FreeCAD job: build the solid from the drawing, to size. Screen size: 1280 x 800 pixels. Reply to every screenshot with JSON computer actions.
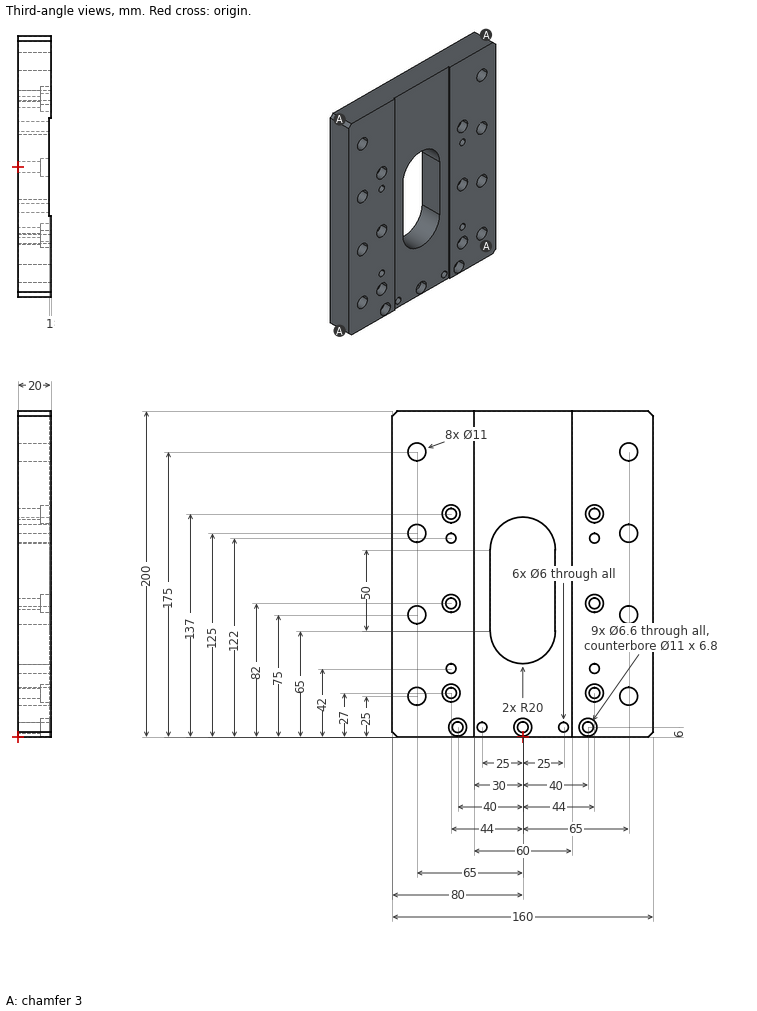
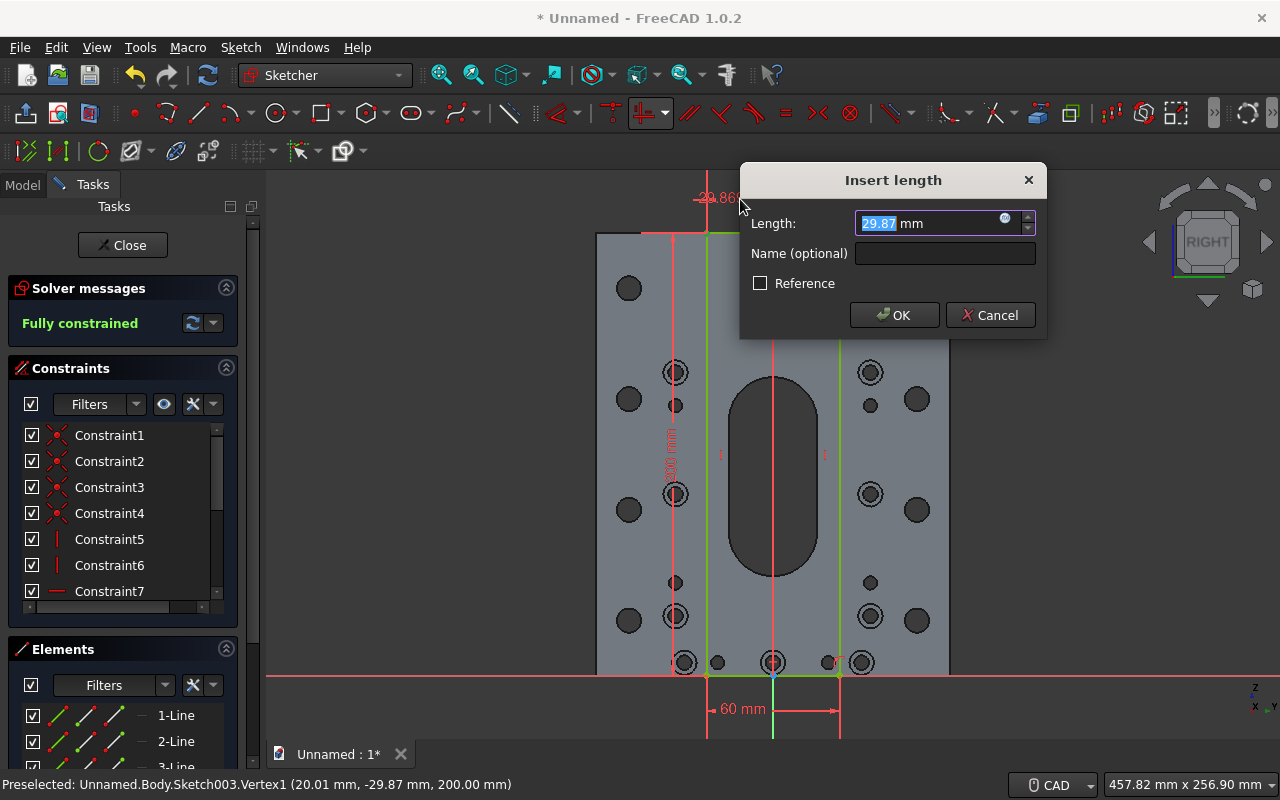
{"action": "type", "text": "30"}
{"action": "key", "text": "Return"}
{"action": "key", "text": "Escape"}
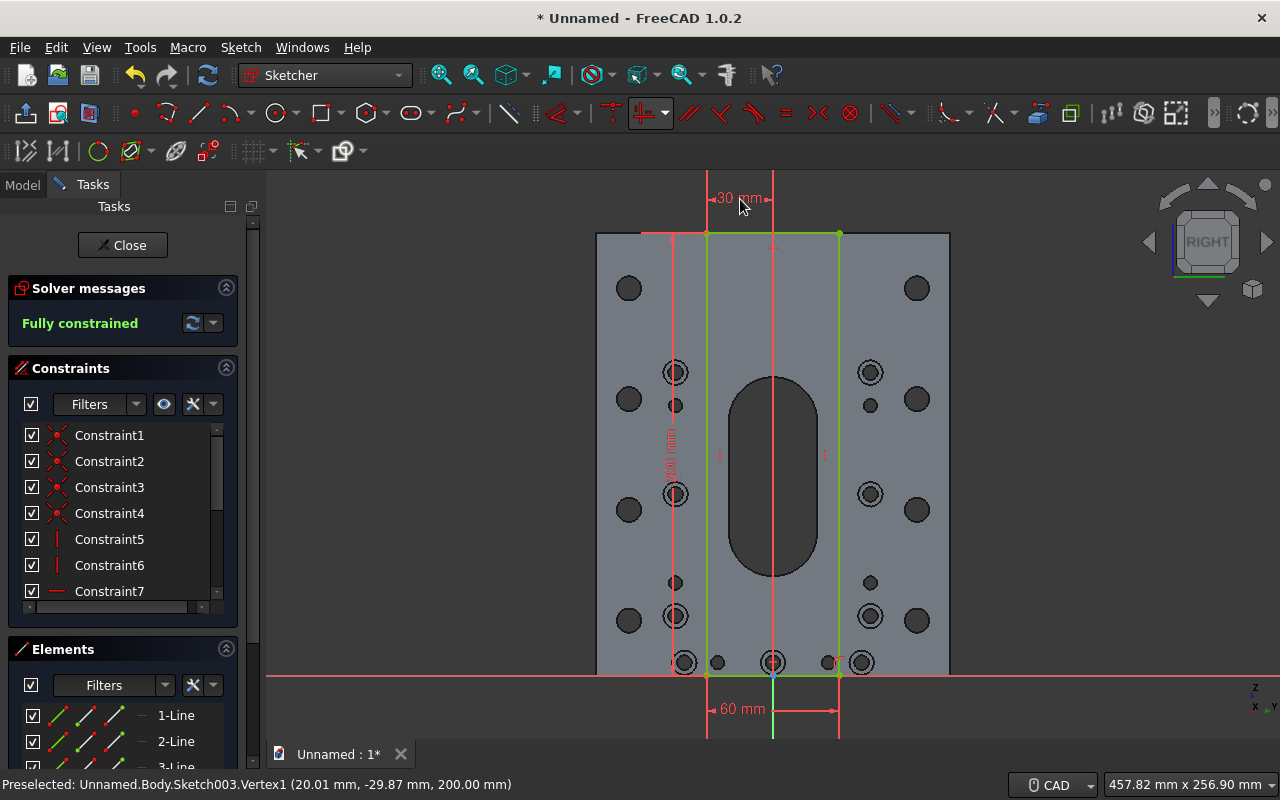
{"action": "left_click", "coordinate": [123, 245]}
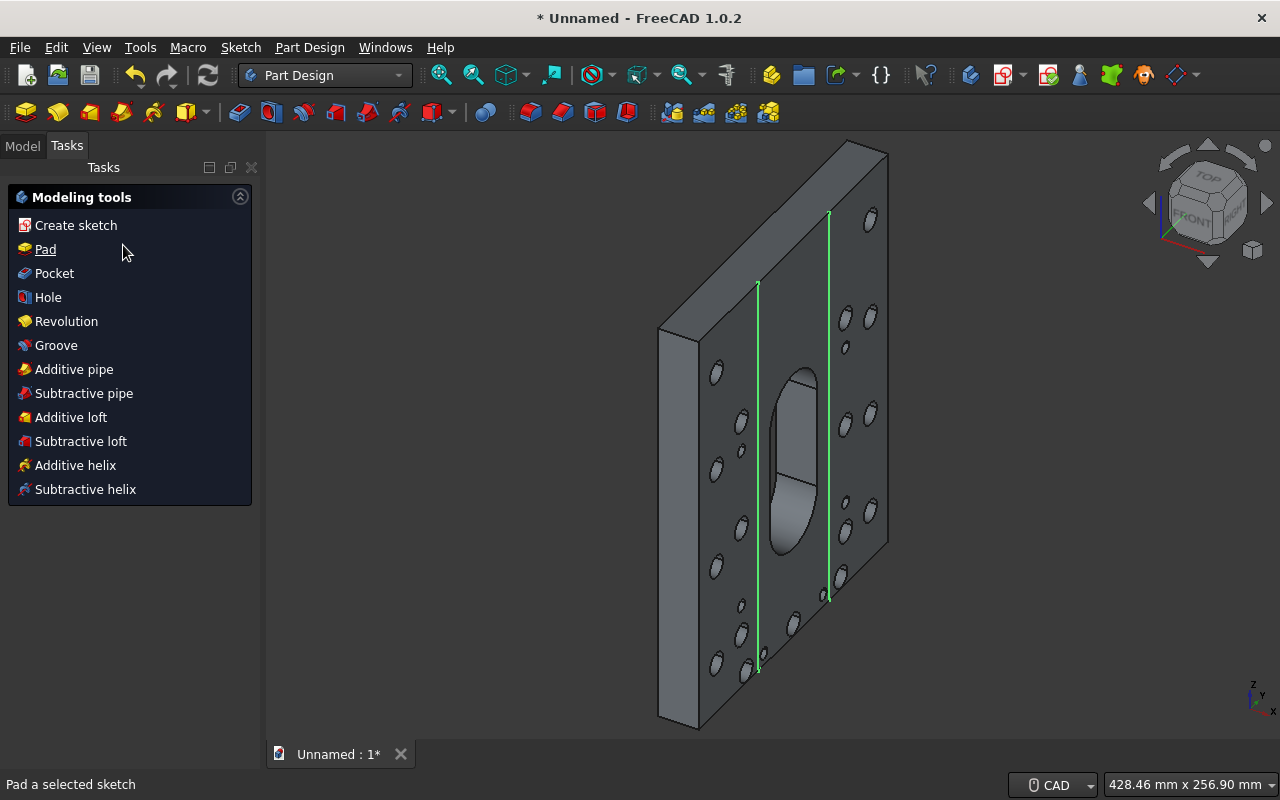
{"action": "left_click", "coordinate": [240, 112]}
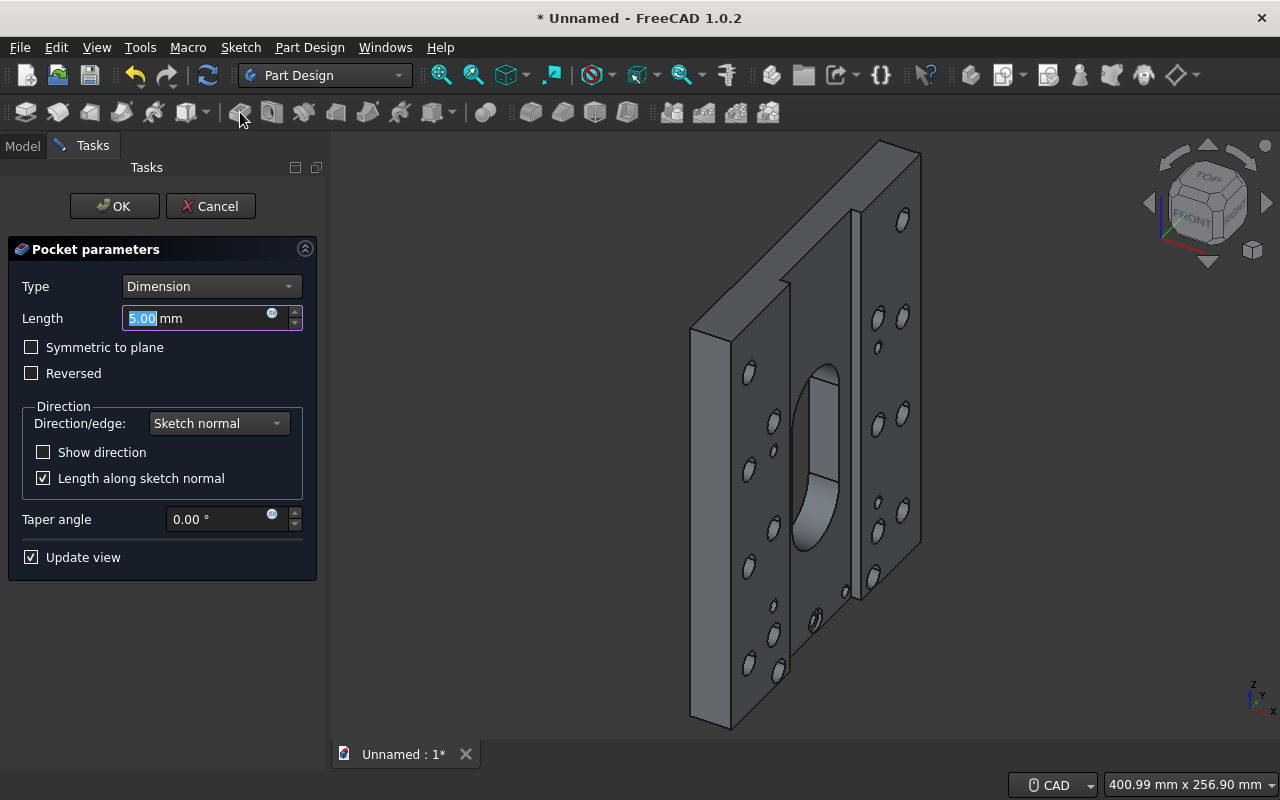
{"action": "type", "text": "1"}
{"action": "key", "text": "Tab"}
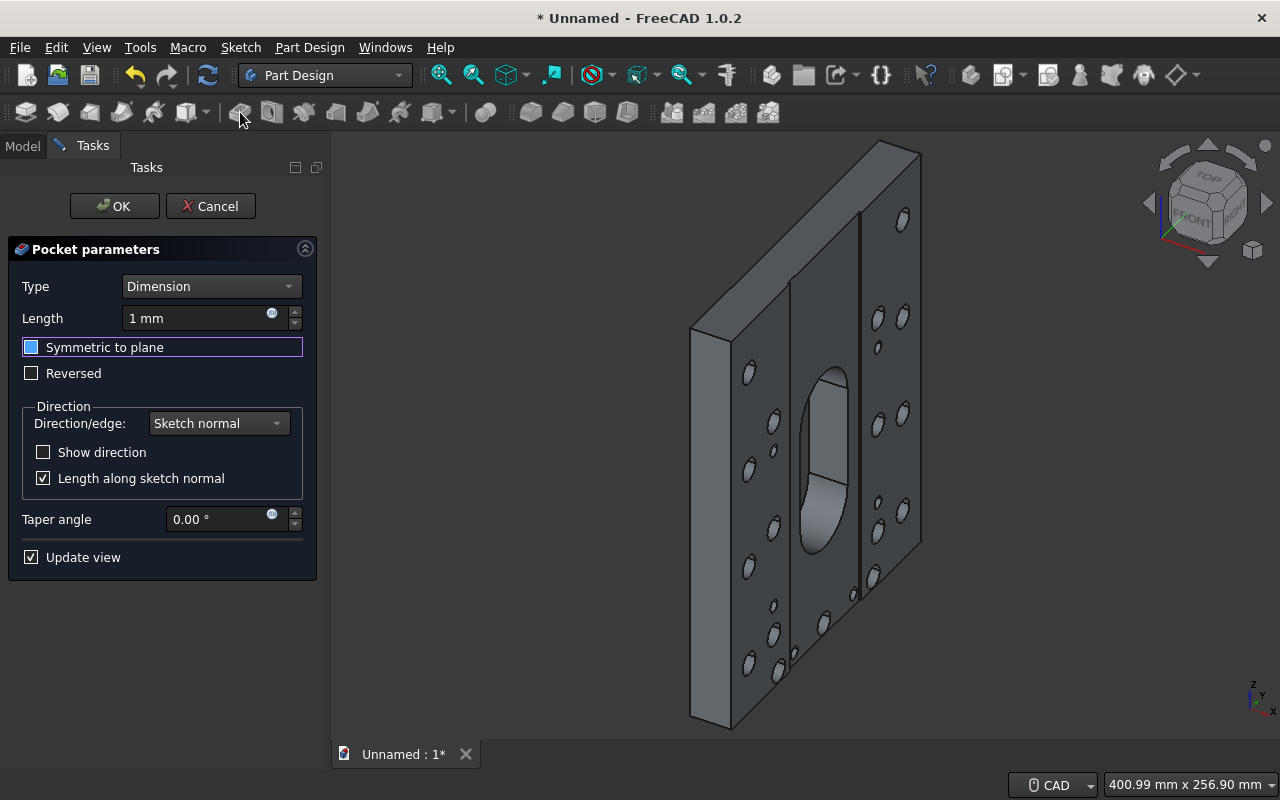
{"action": "left_click", "coordinate": [115, 206]}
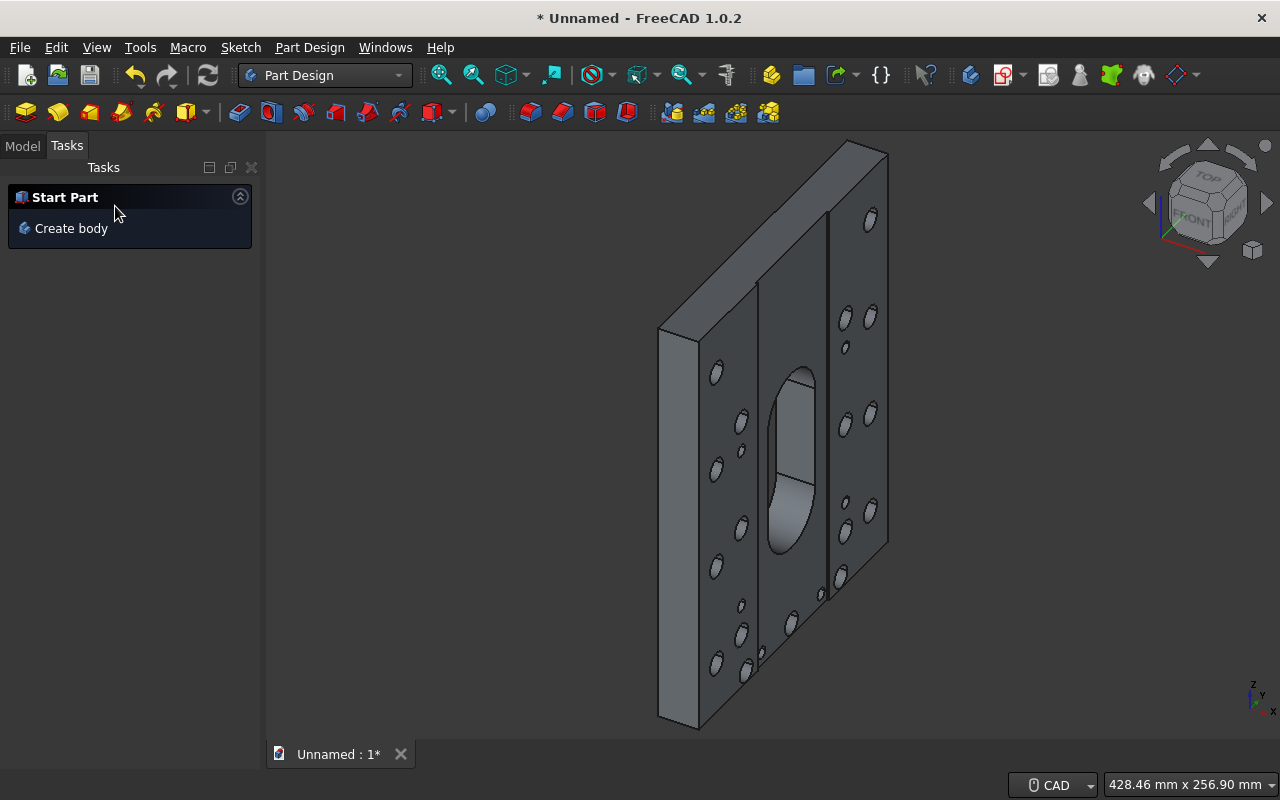
{"action": "left_click", "coordinate": [678, 334]}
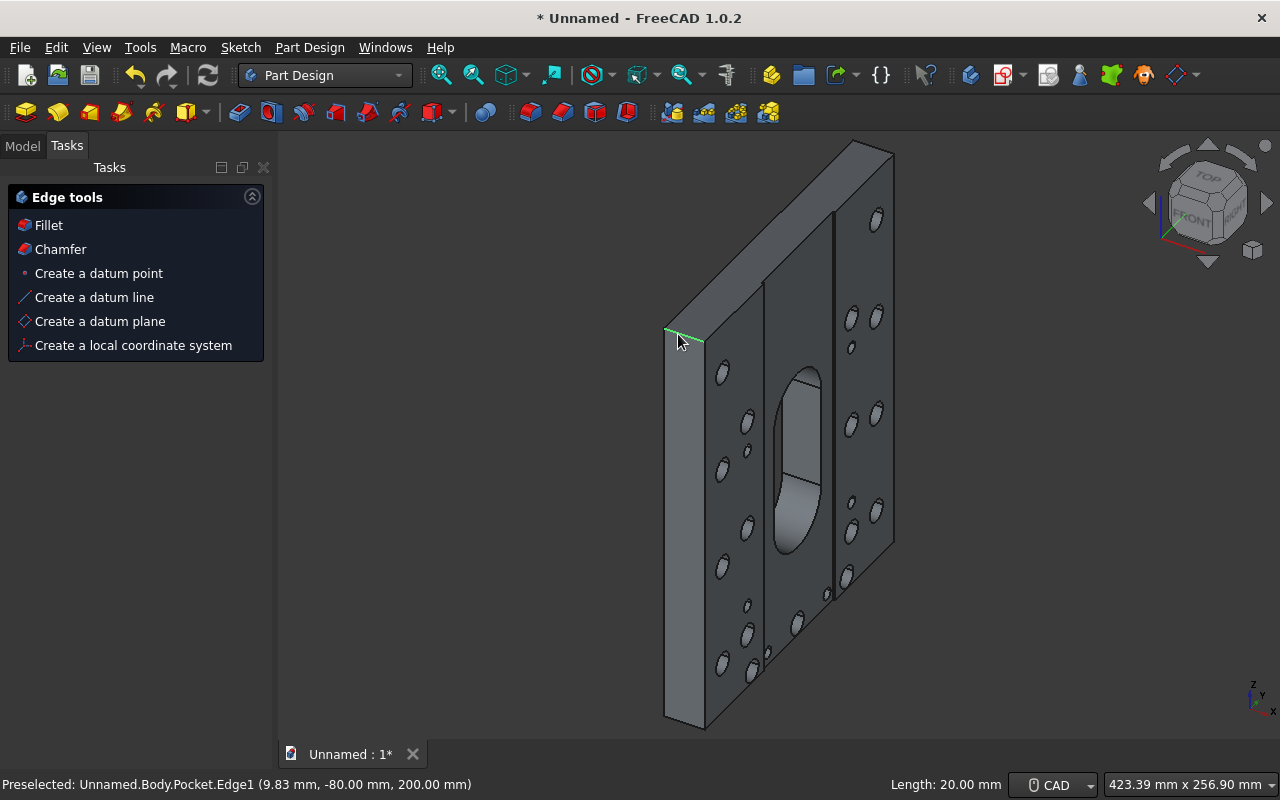
{"action": "key", "text": "0"}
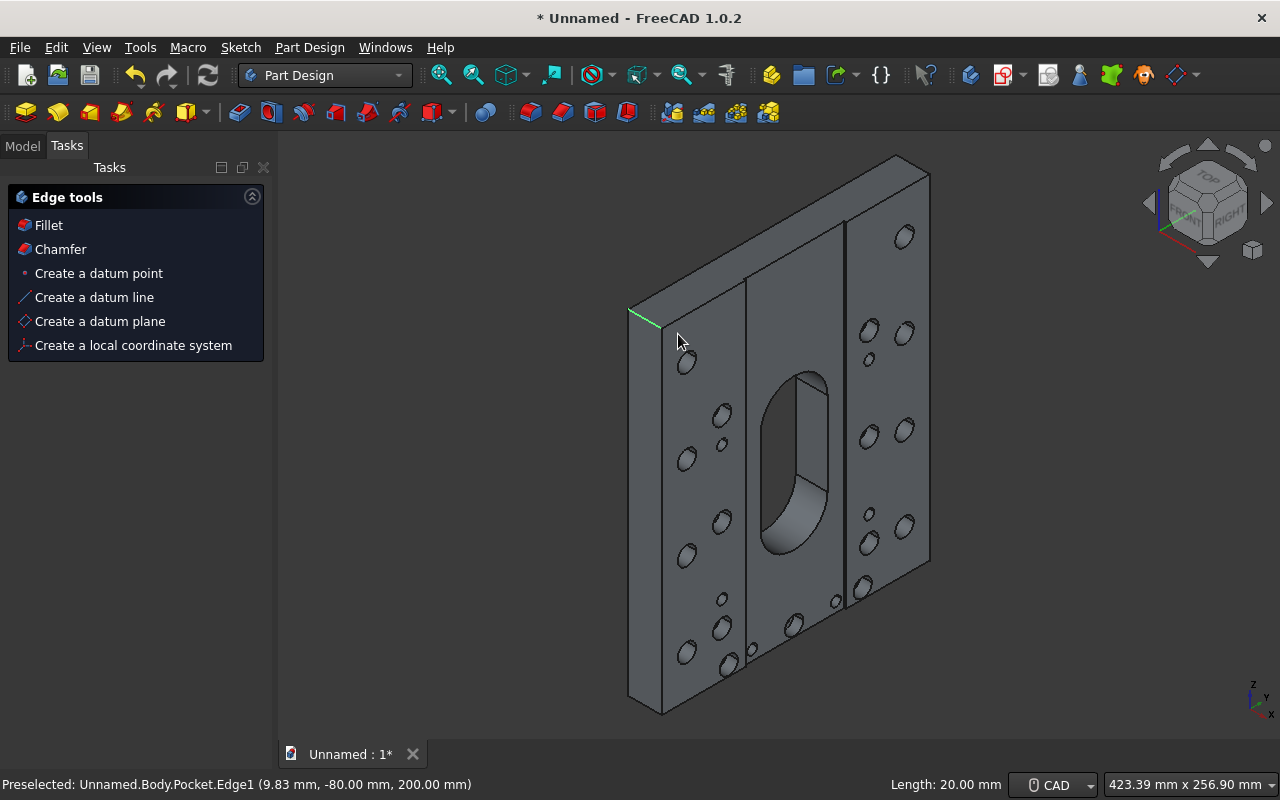
{"action": "key", "text": "2"}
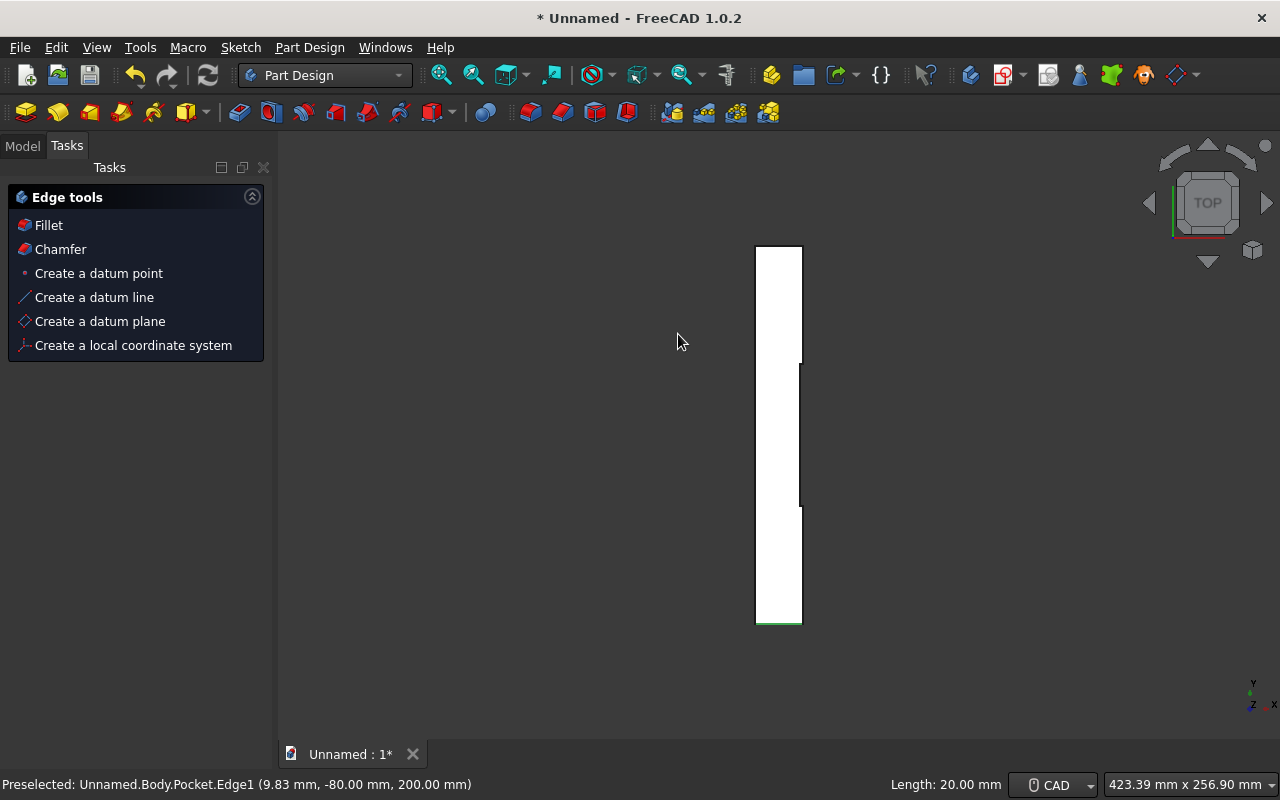
{"action": "left_click", "coordinate": [779, 245], "text": "ctrl"}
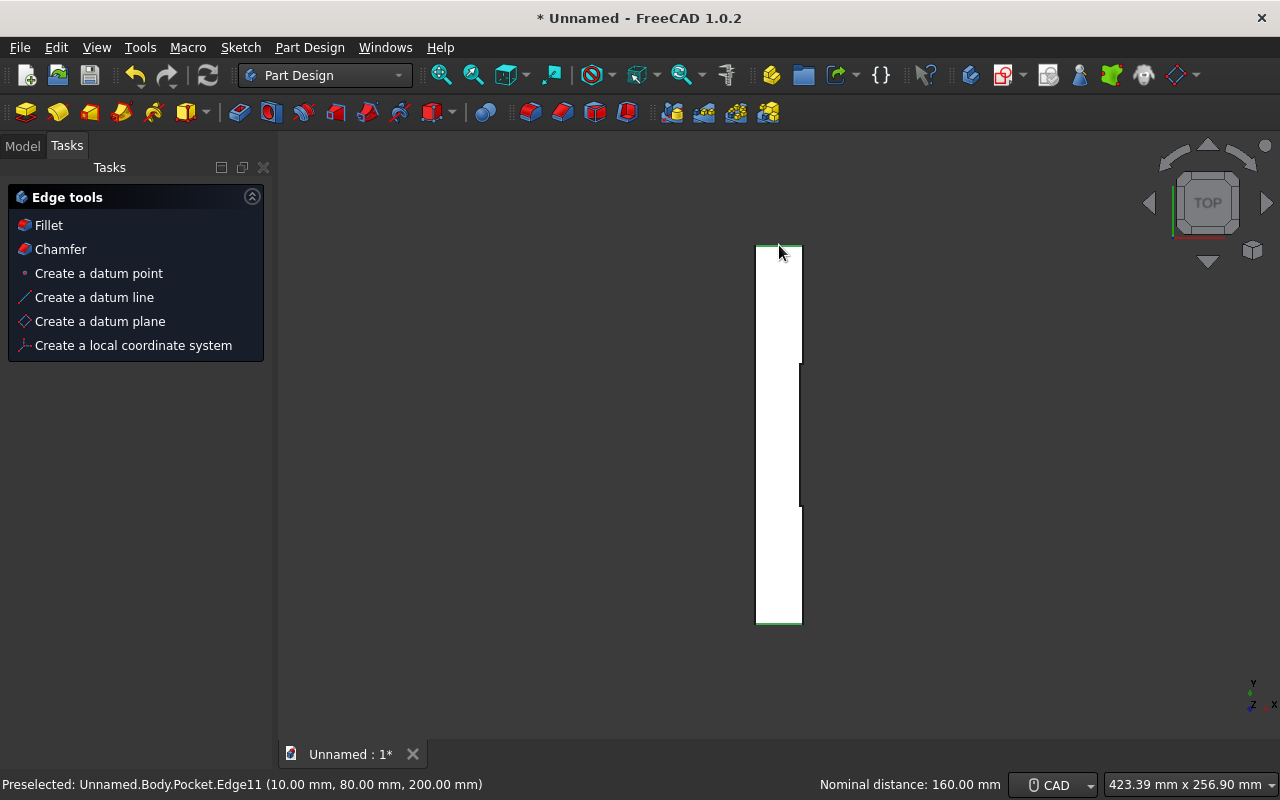
{"action": "key", "text": "1"}